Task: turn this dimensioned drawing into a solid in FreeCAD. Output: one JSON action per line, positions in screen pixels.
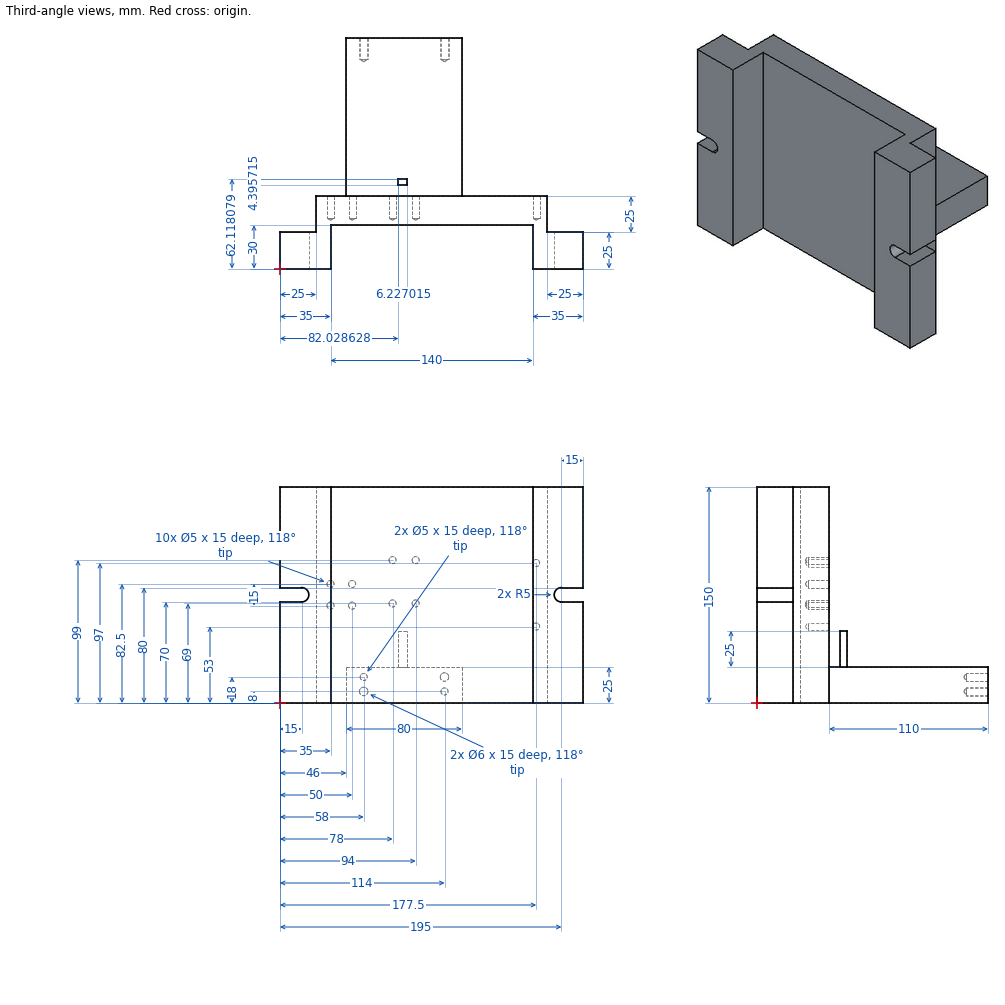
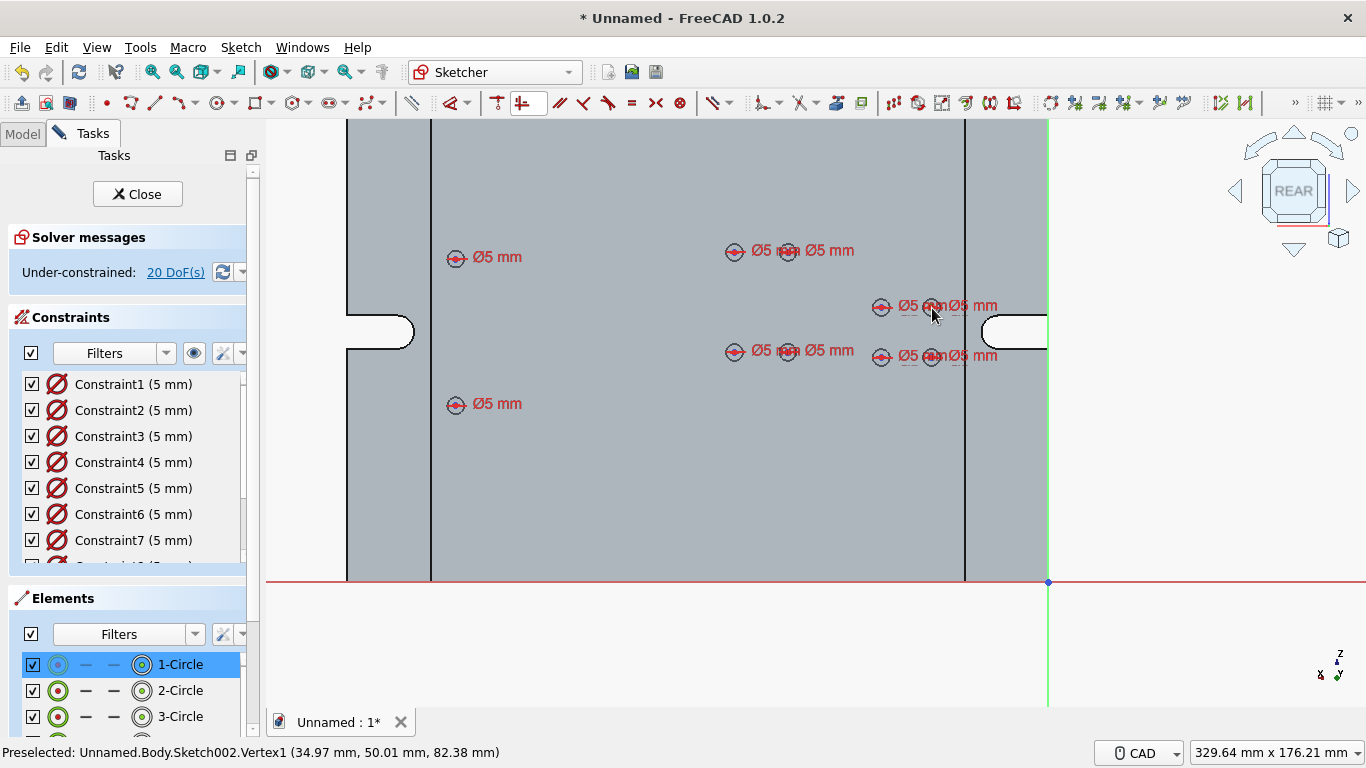
{"action": "left_click", "coordinate": [932, 358]}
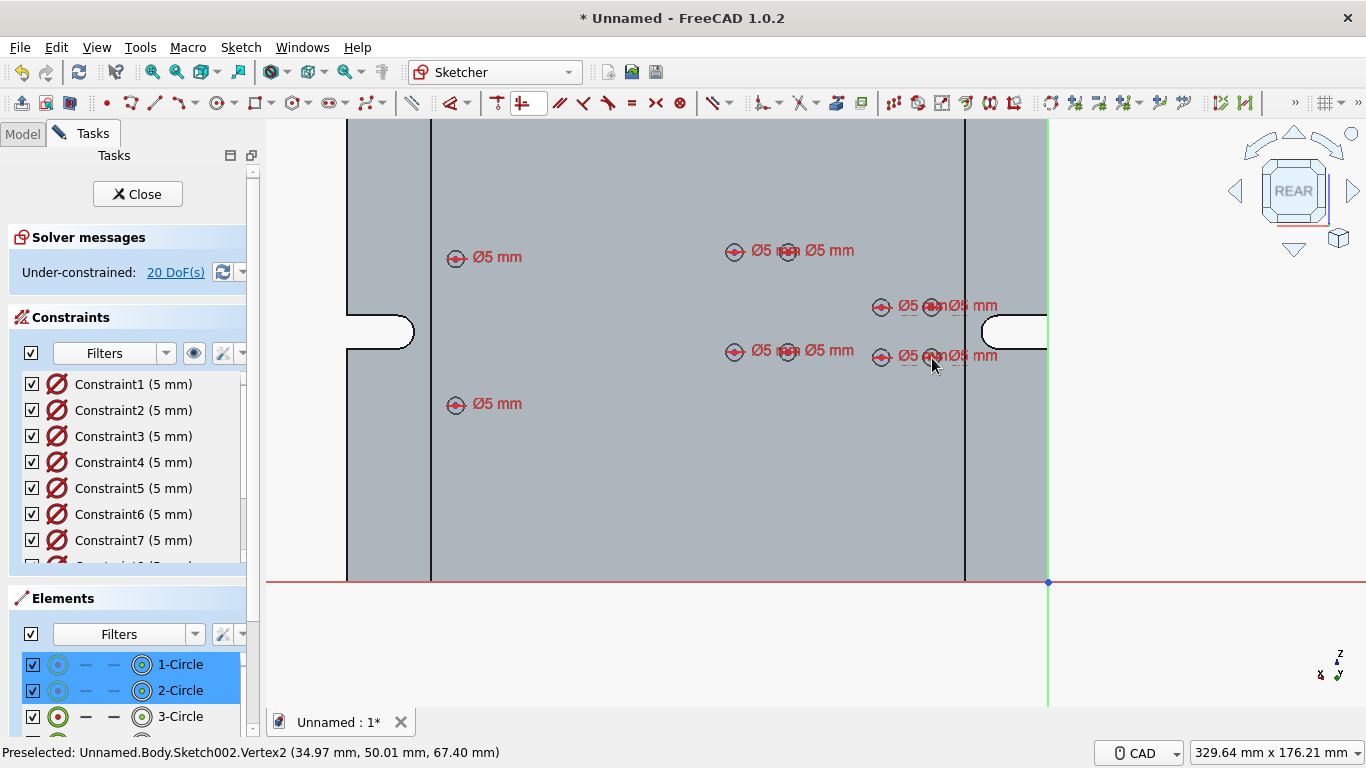
{"action": "key", "text": "v"}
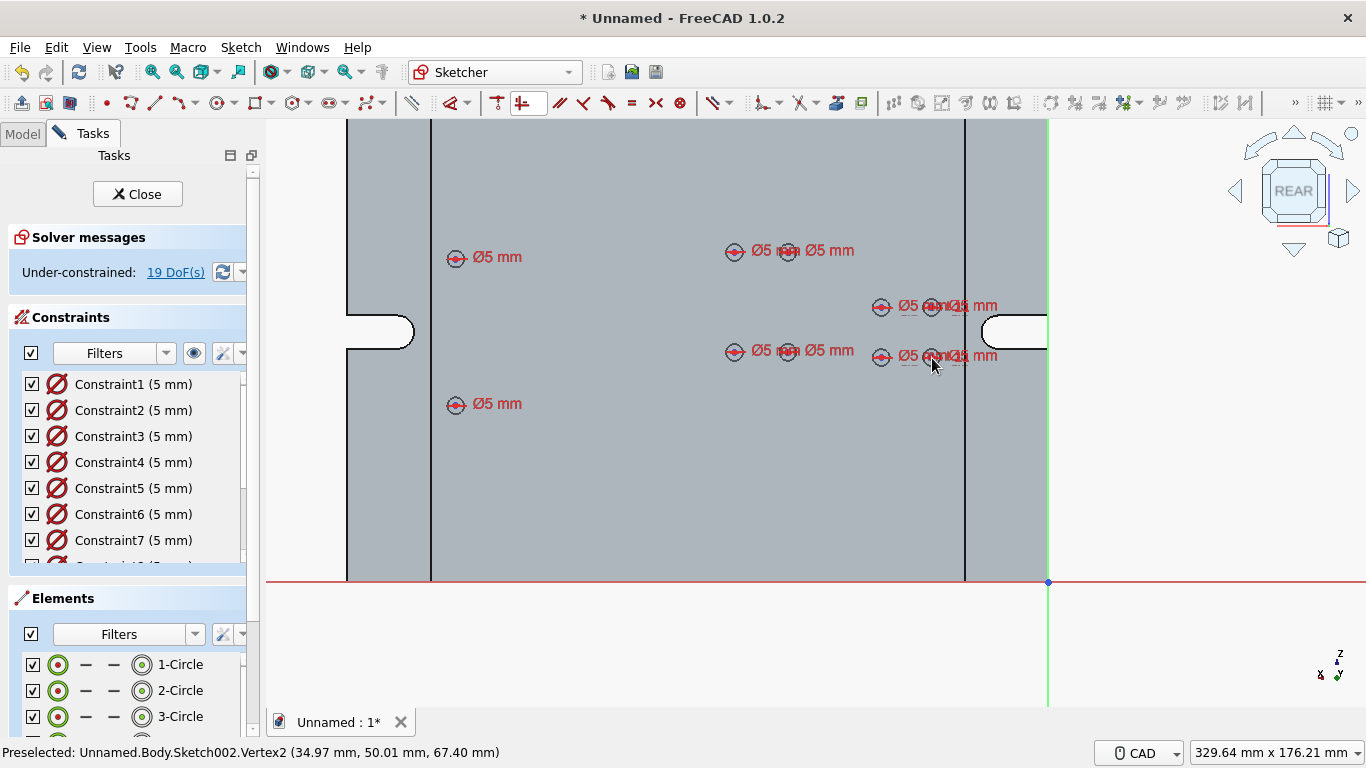
{"action": "left_click", "coordinate": [932, 358]}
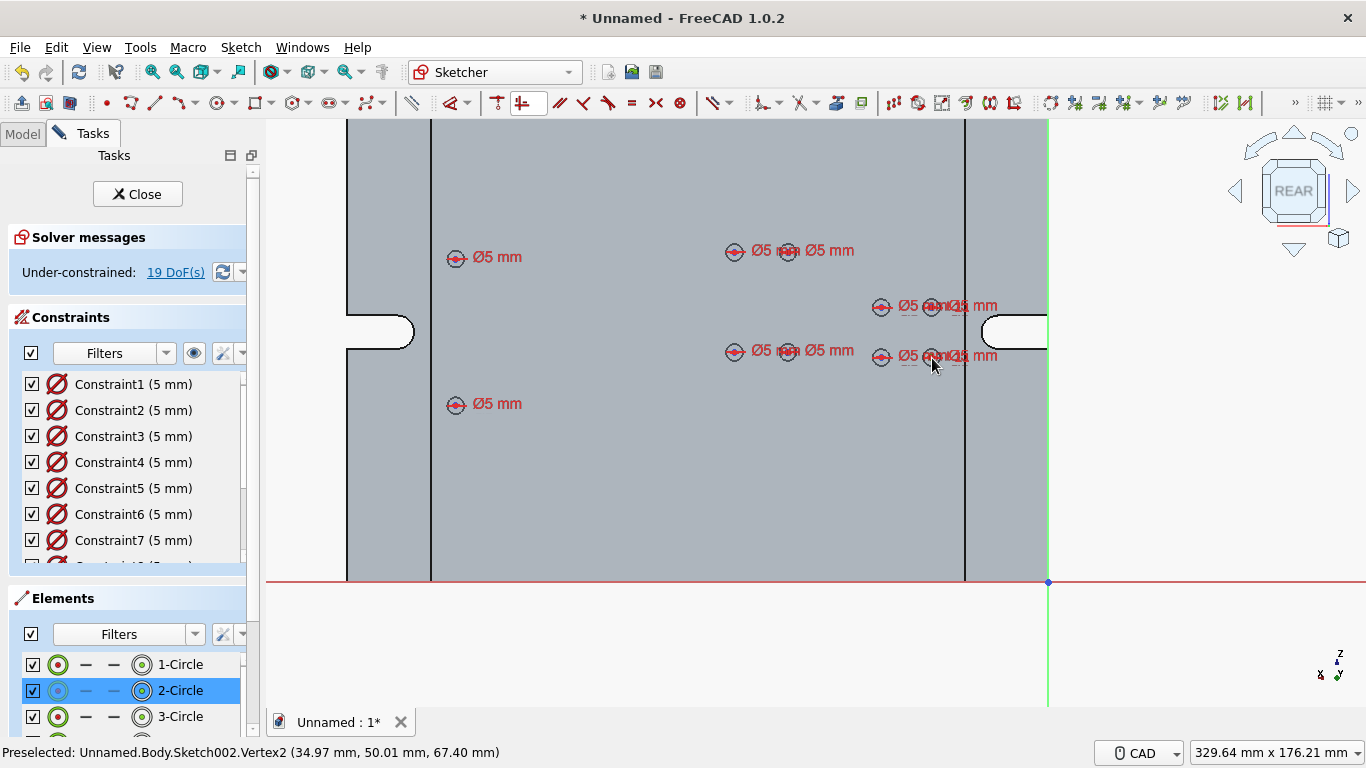
{"action": "left_click", "coordinate": [881, 358]}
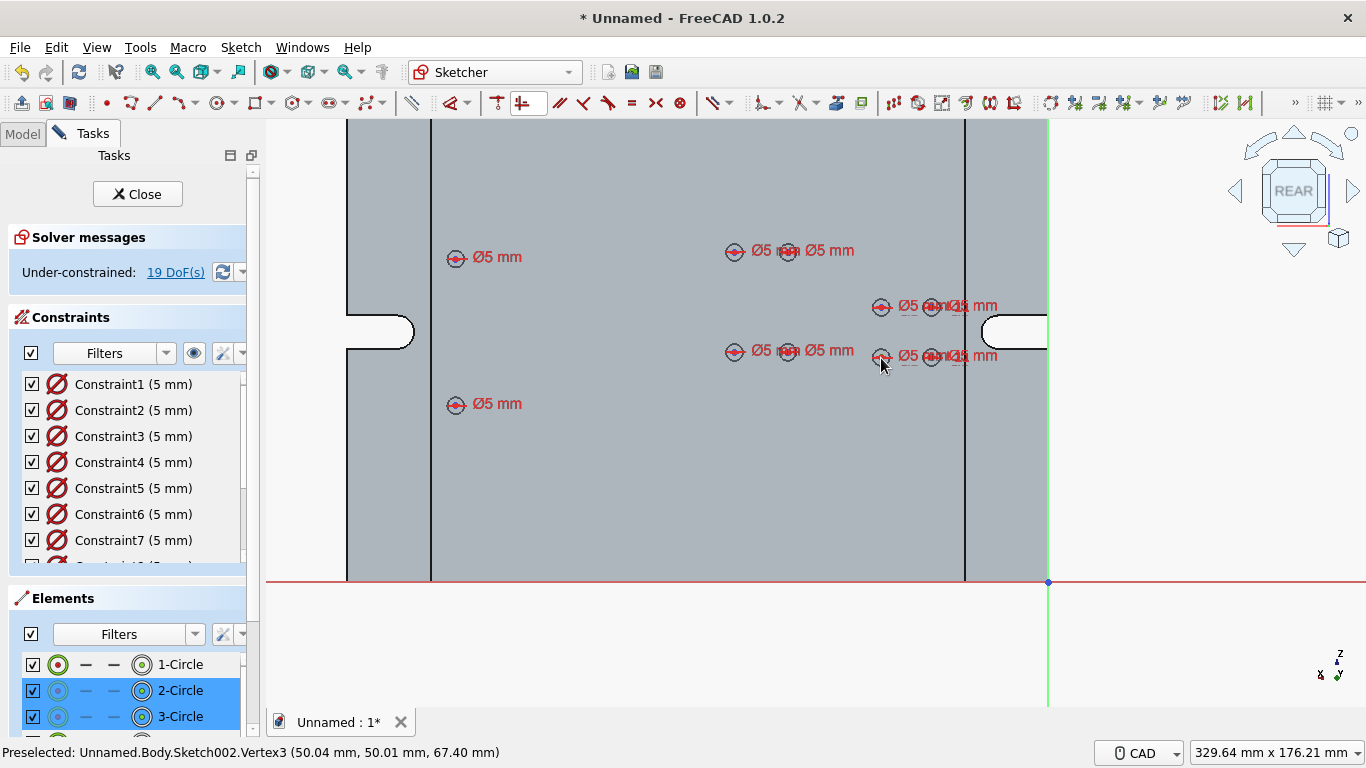
{"action": "left_click", "coordinate": [542, 104]}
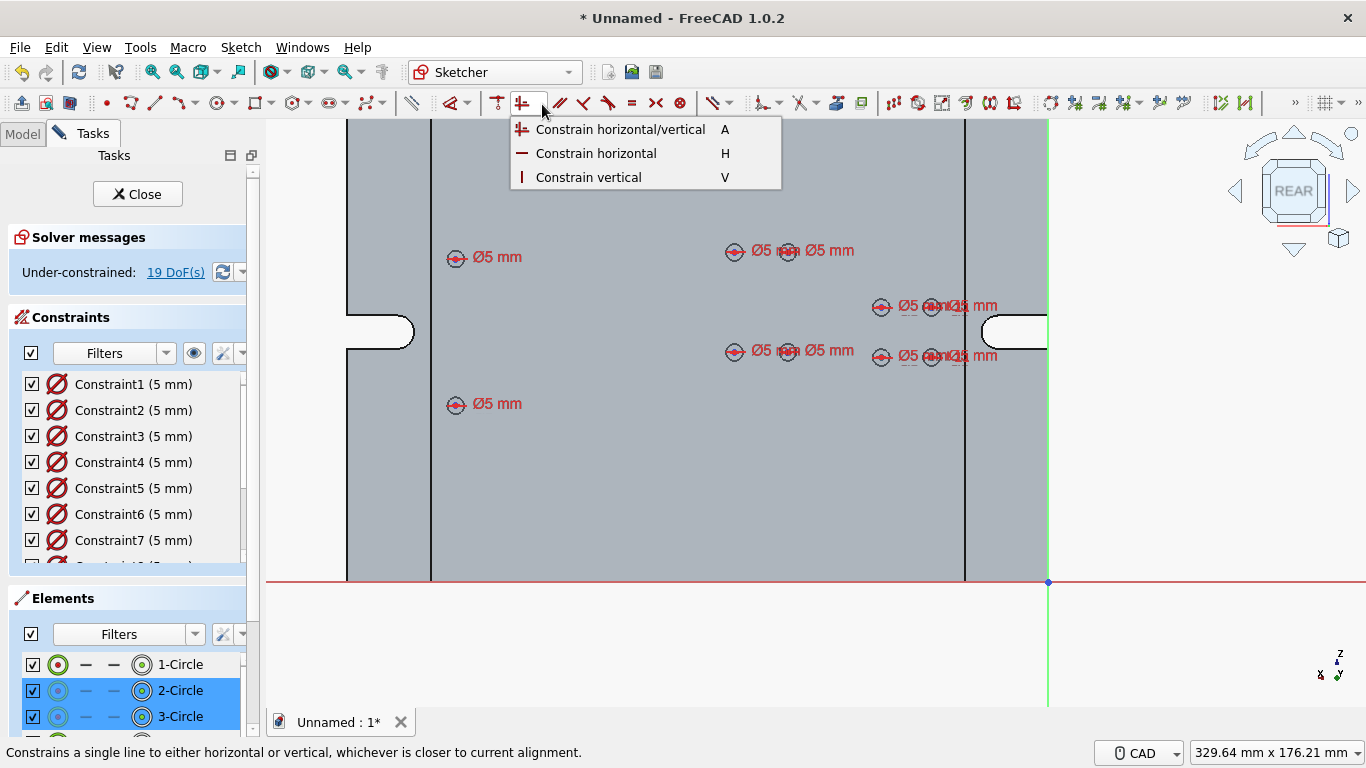
{"action": "left_click", "coordinate": [646, 153]}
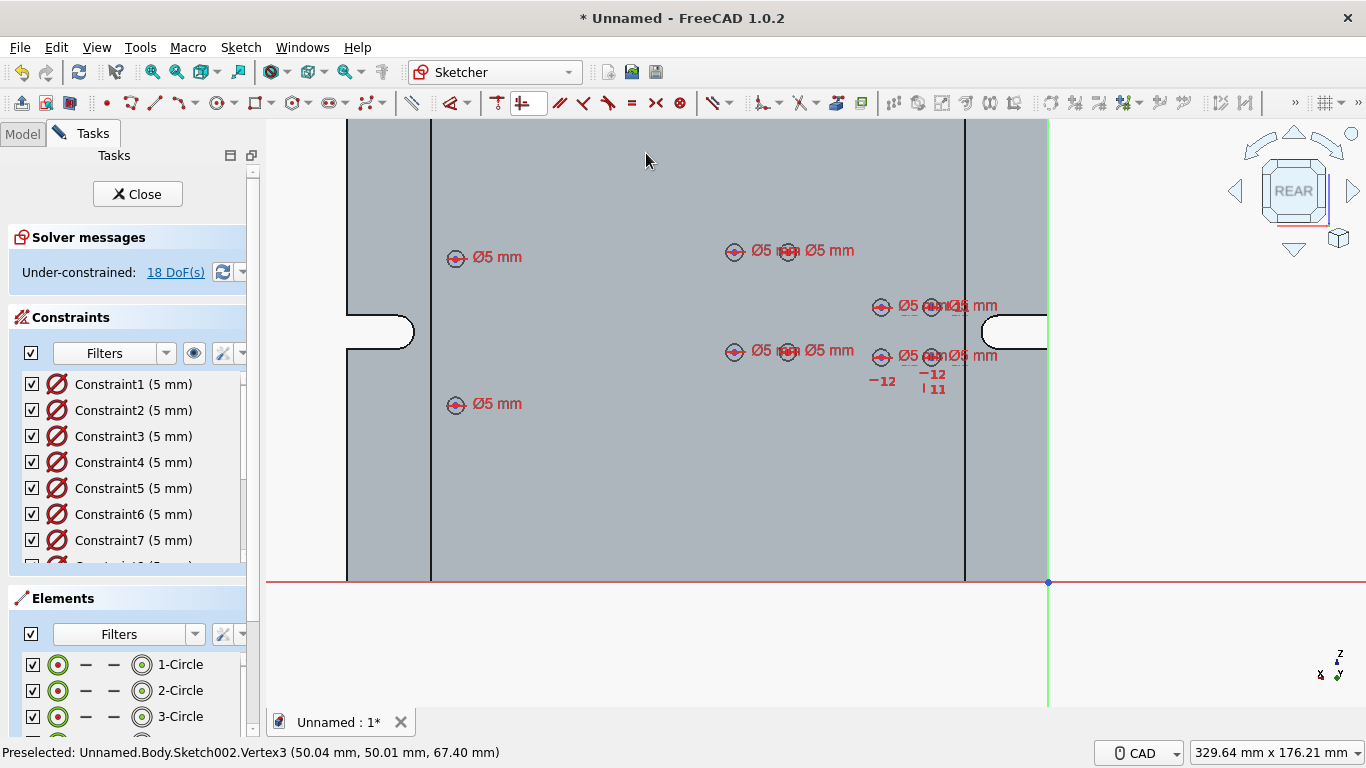
{"action": "left_click", "coordinate": [881, 358]}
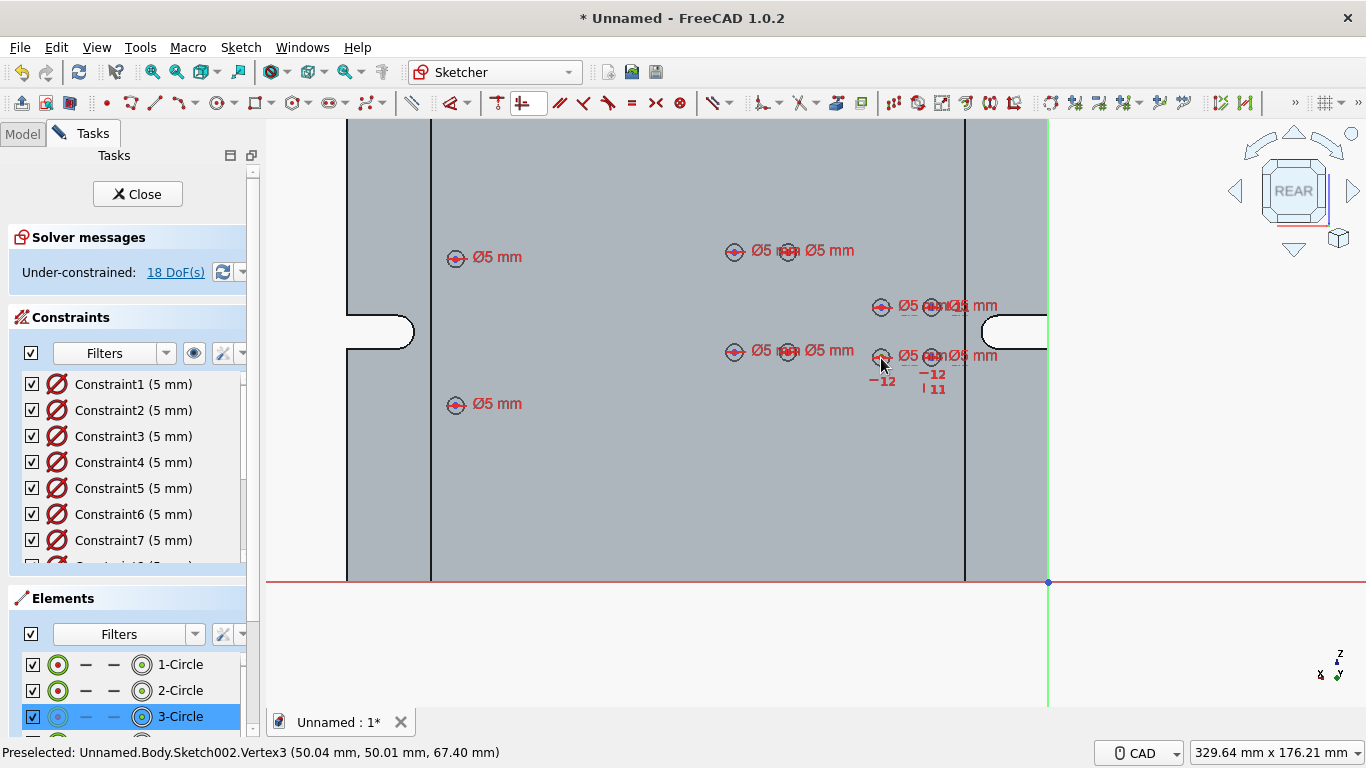
{"action": "left_click", "coordinate": [881, 308]}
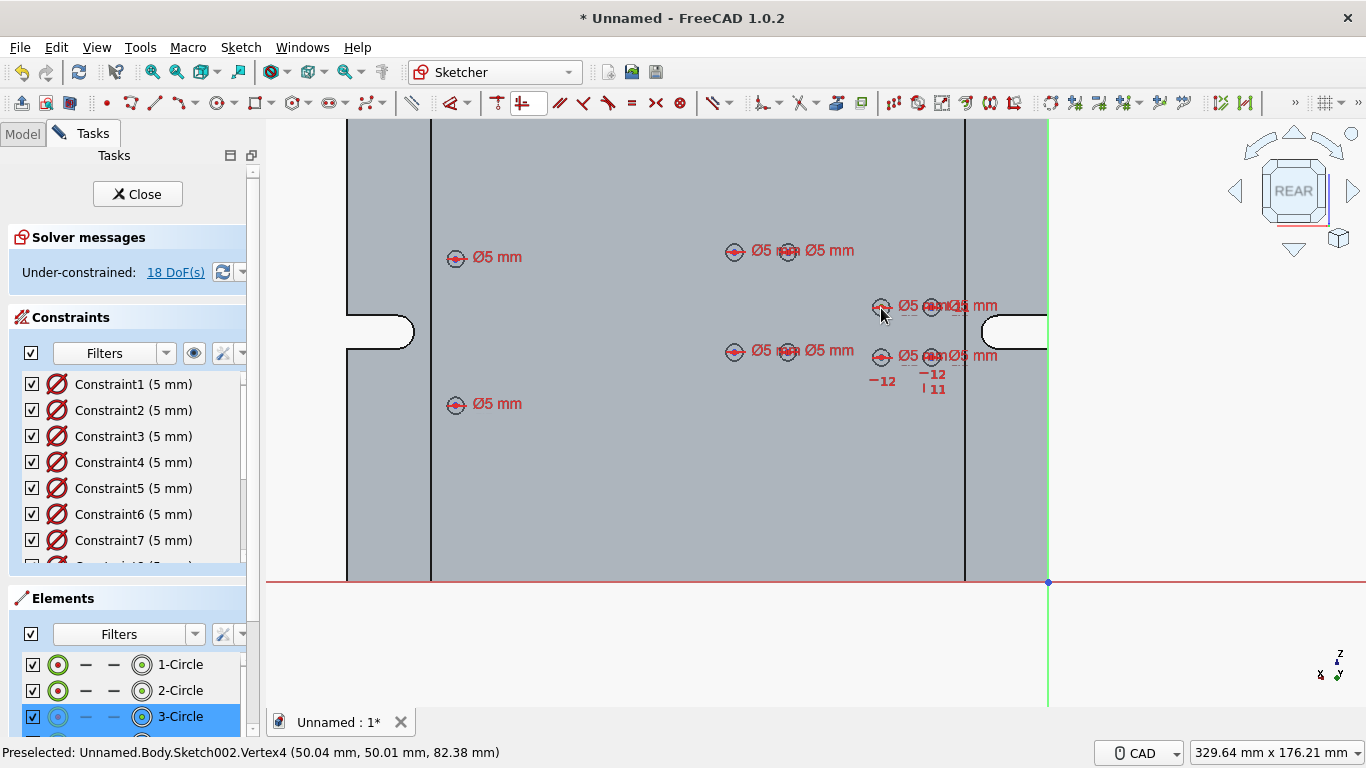
{"action": "left_click", "coordinate": [542, 104]}